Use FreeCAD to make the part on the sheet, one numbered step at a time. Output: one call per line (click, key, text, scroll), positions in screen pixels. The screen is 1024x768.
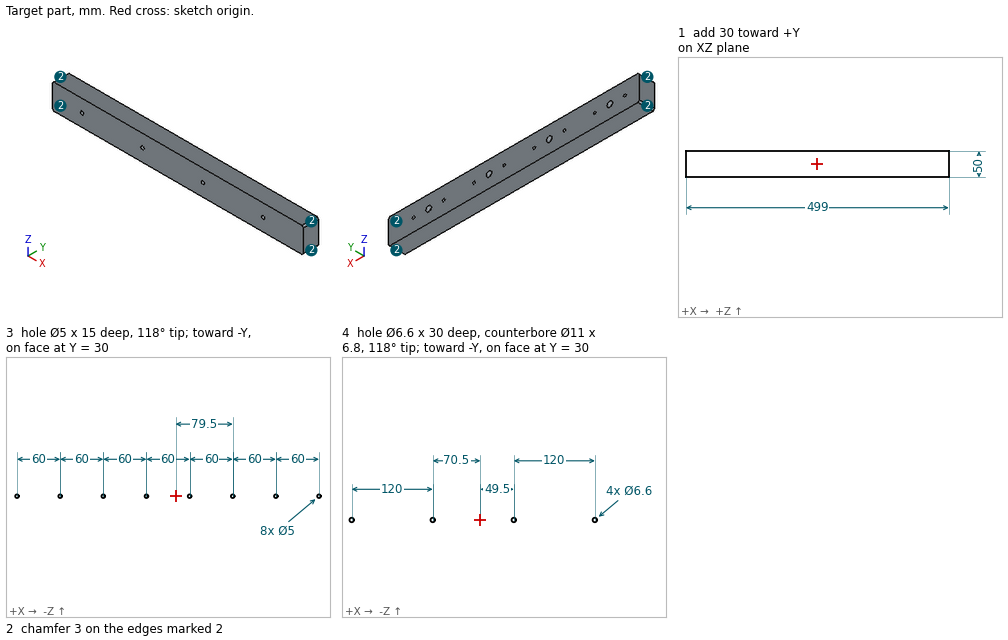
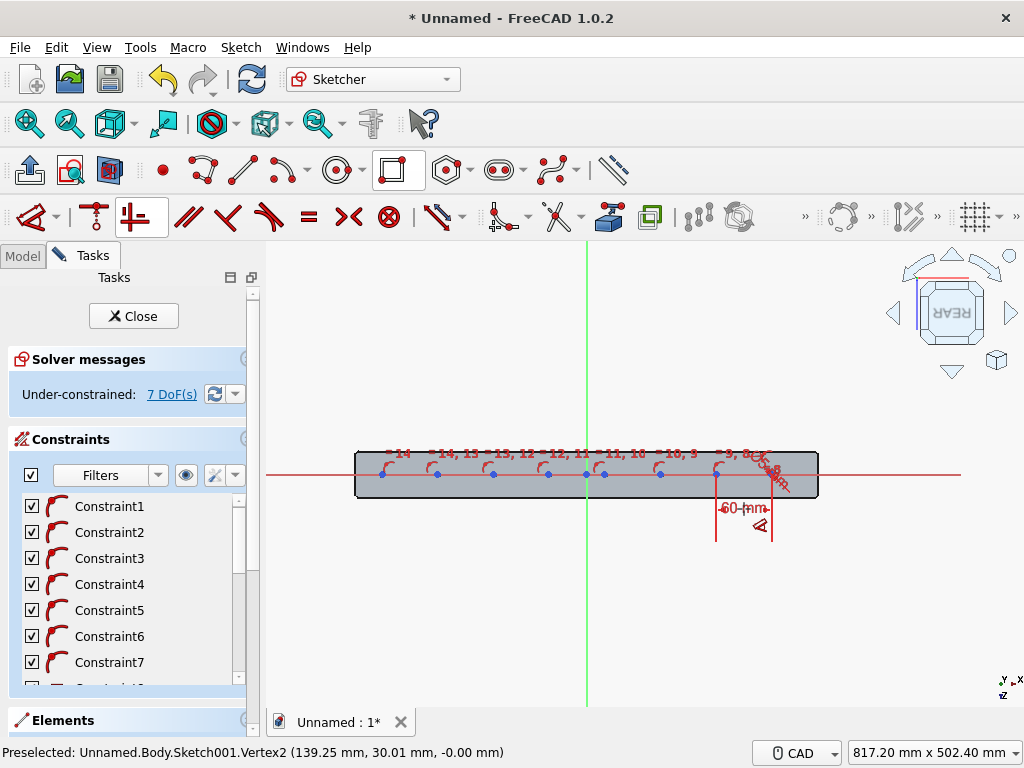
click(716, 475)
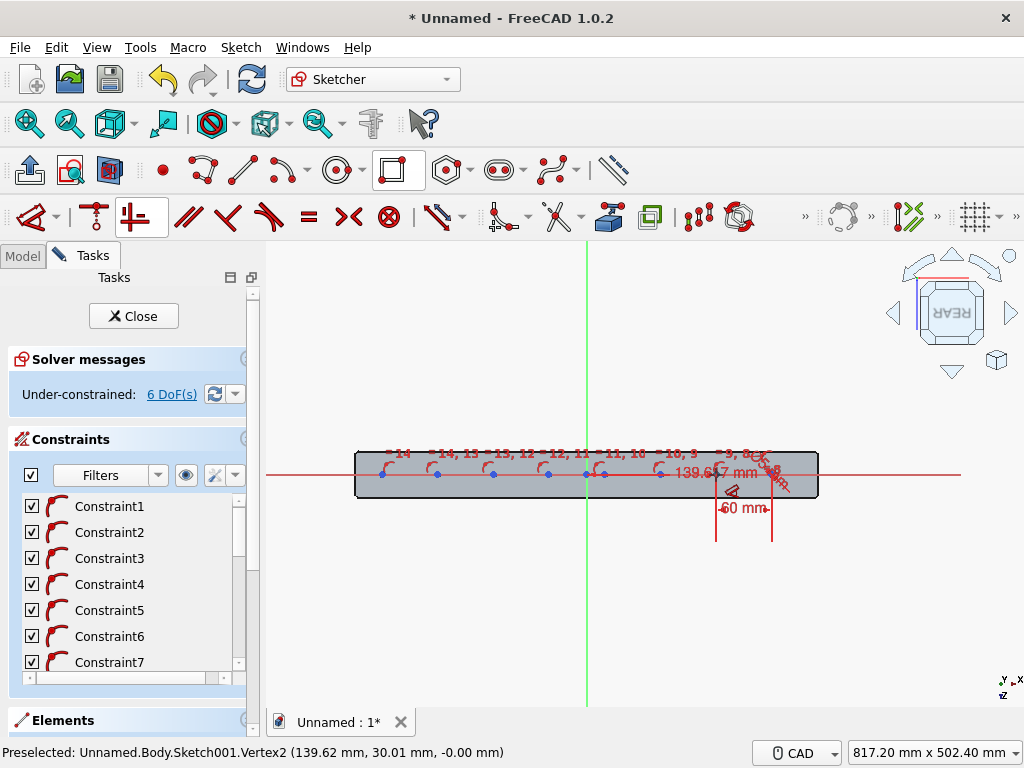
click(661, 475)
click(669, 509)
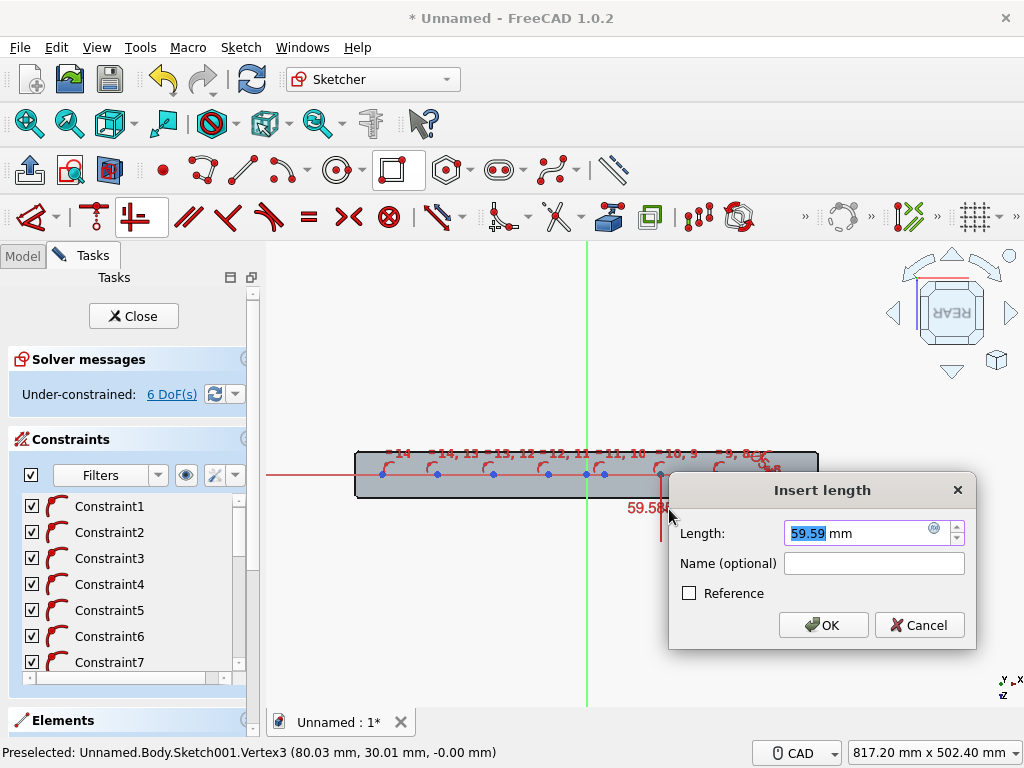
text(60)
key(Return)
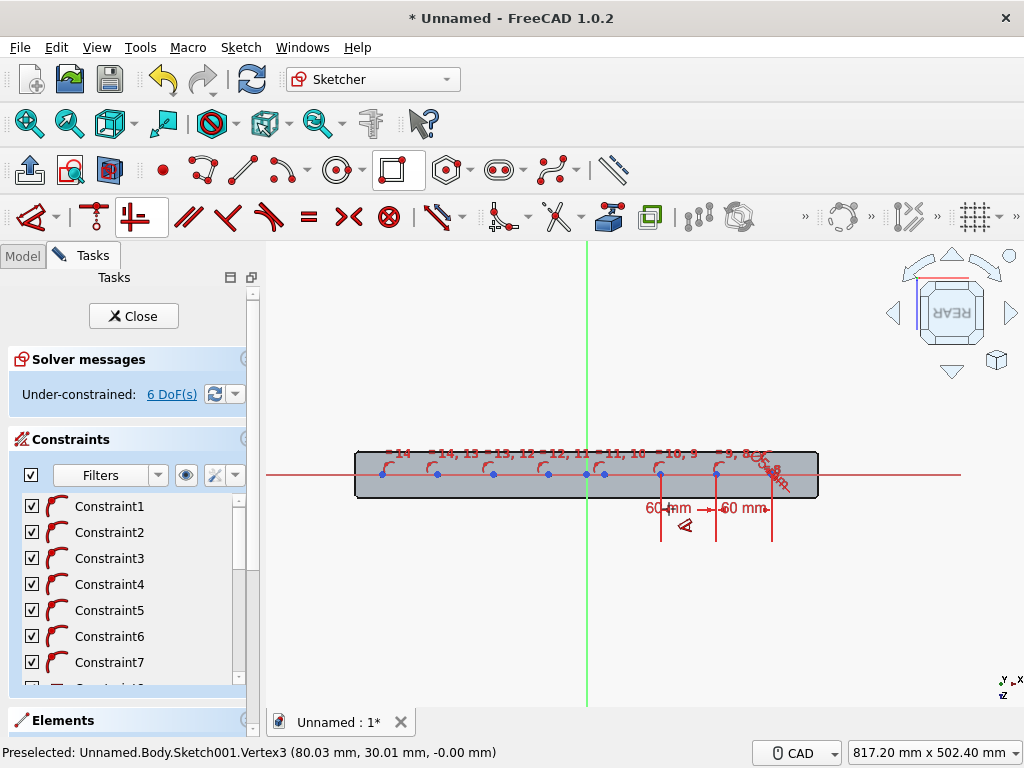
click(661, 475)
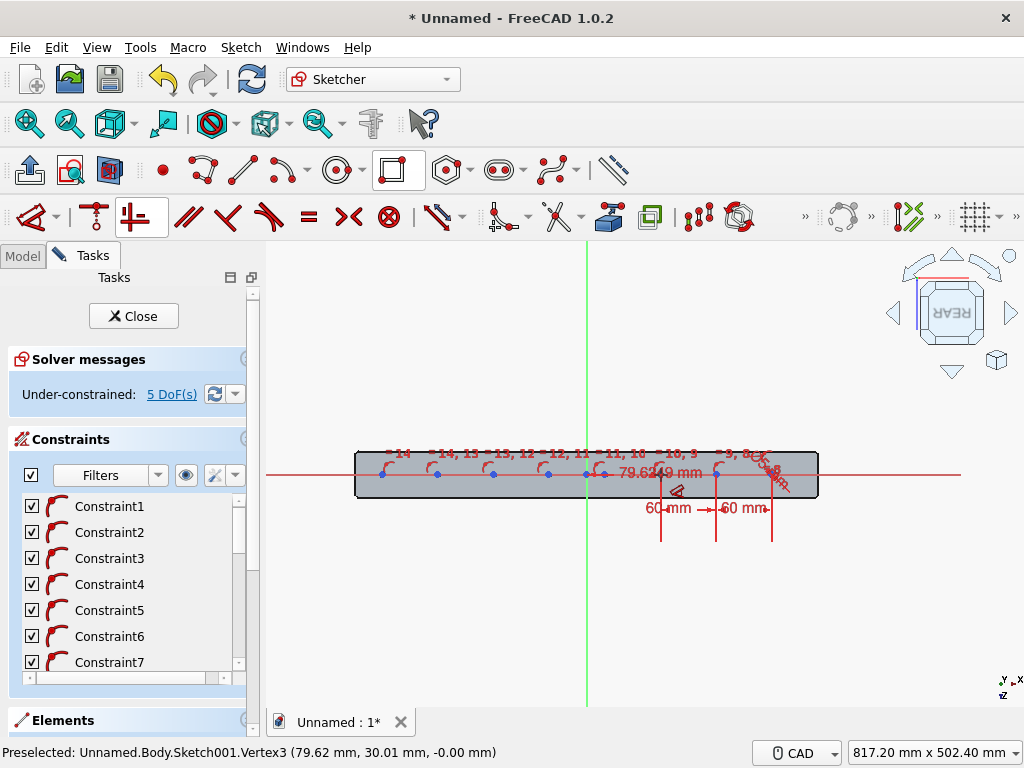
click(605, 475)
click(633, 441)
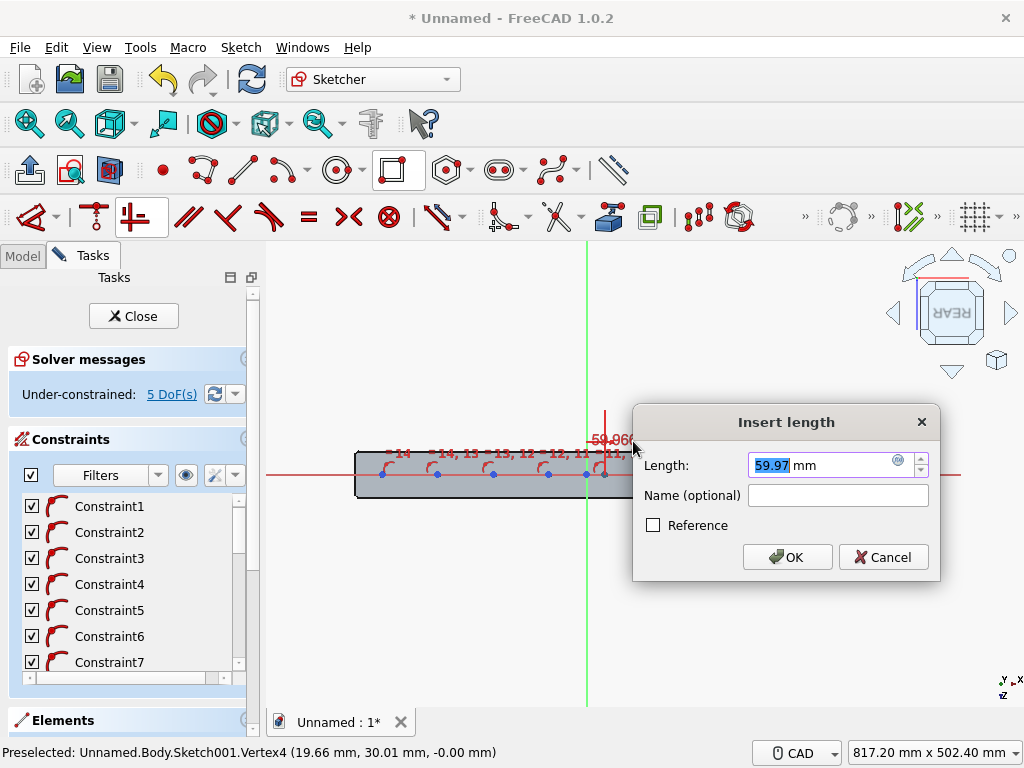
text(60)
key(Return)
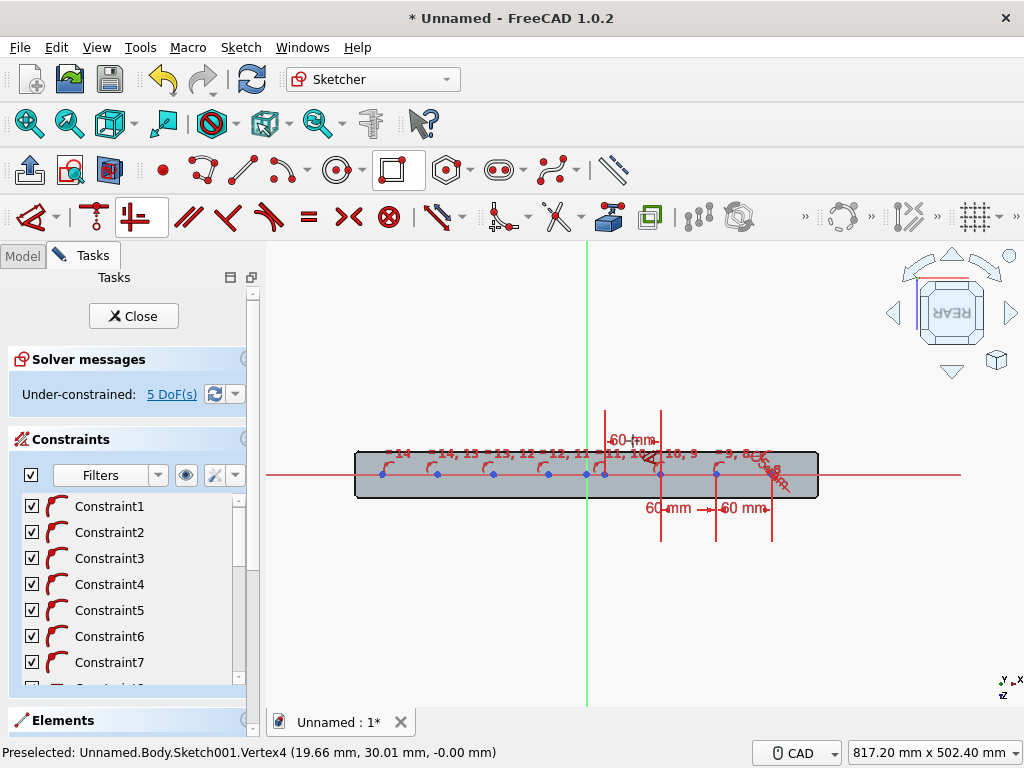
click(605, 475)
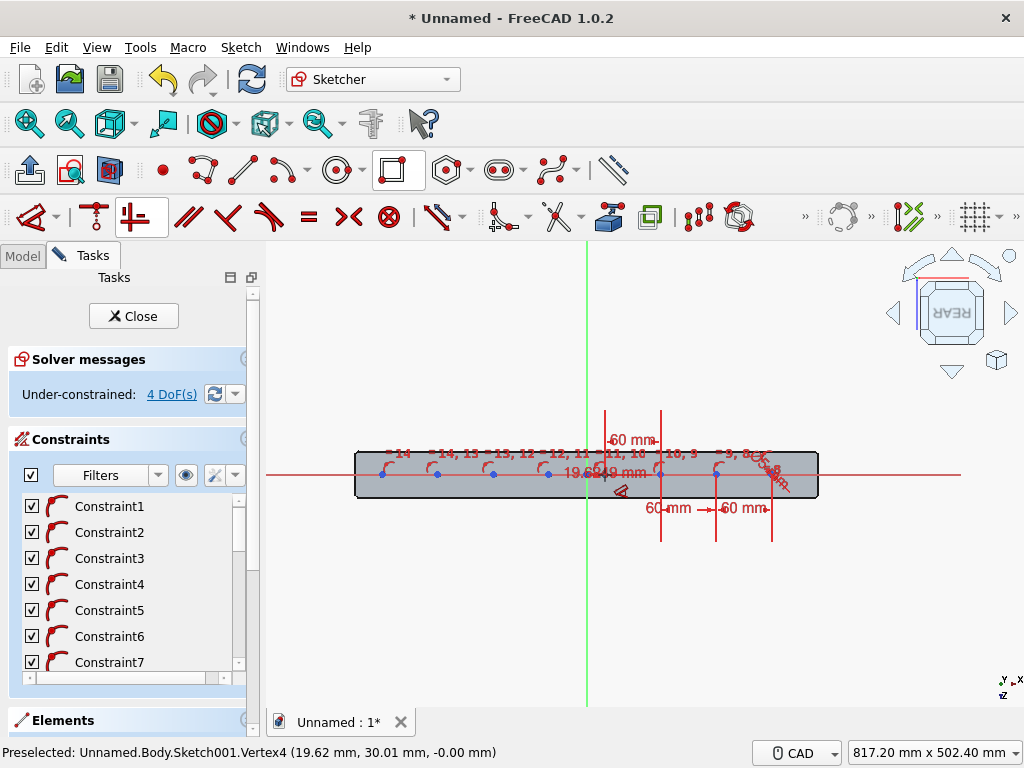
click(549, 475)
click(564, 509)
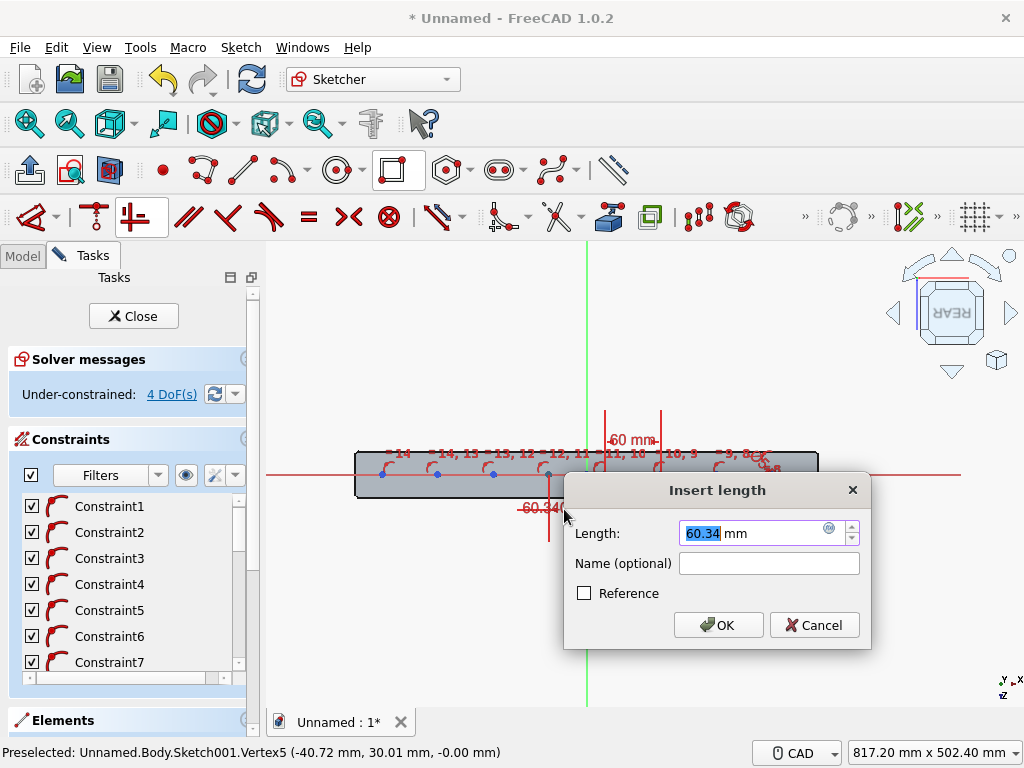
text(60)
key(Return)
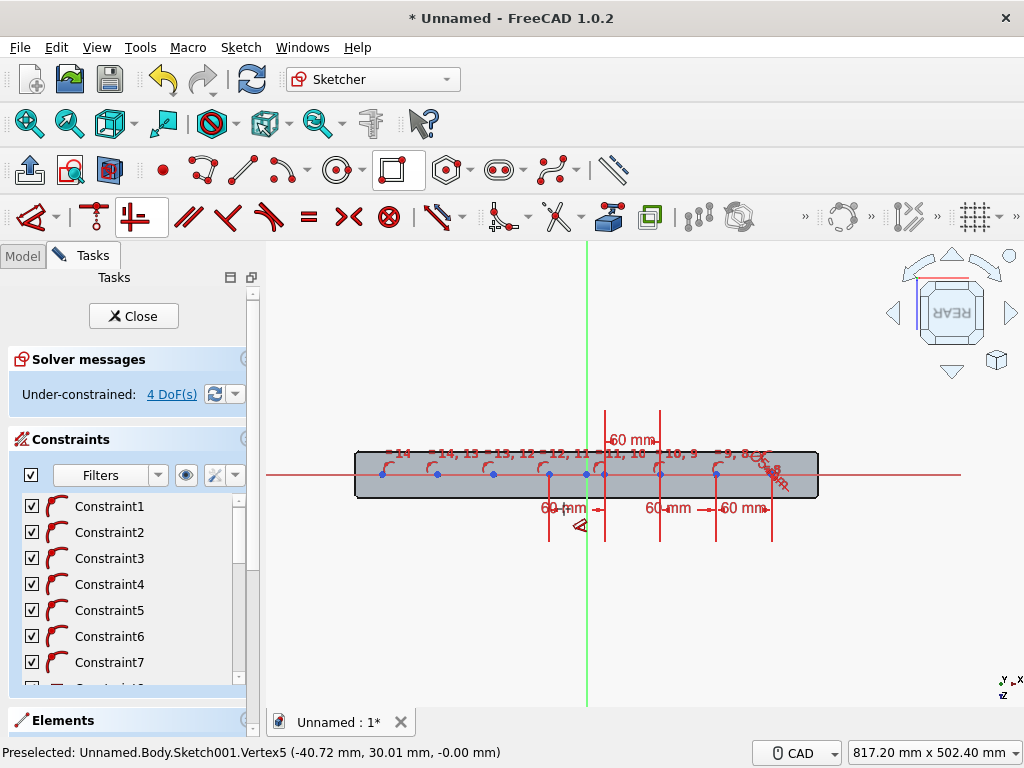
click(549, 475)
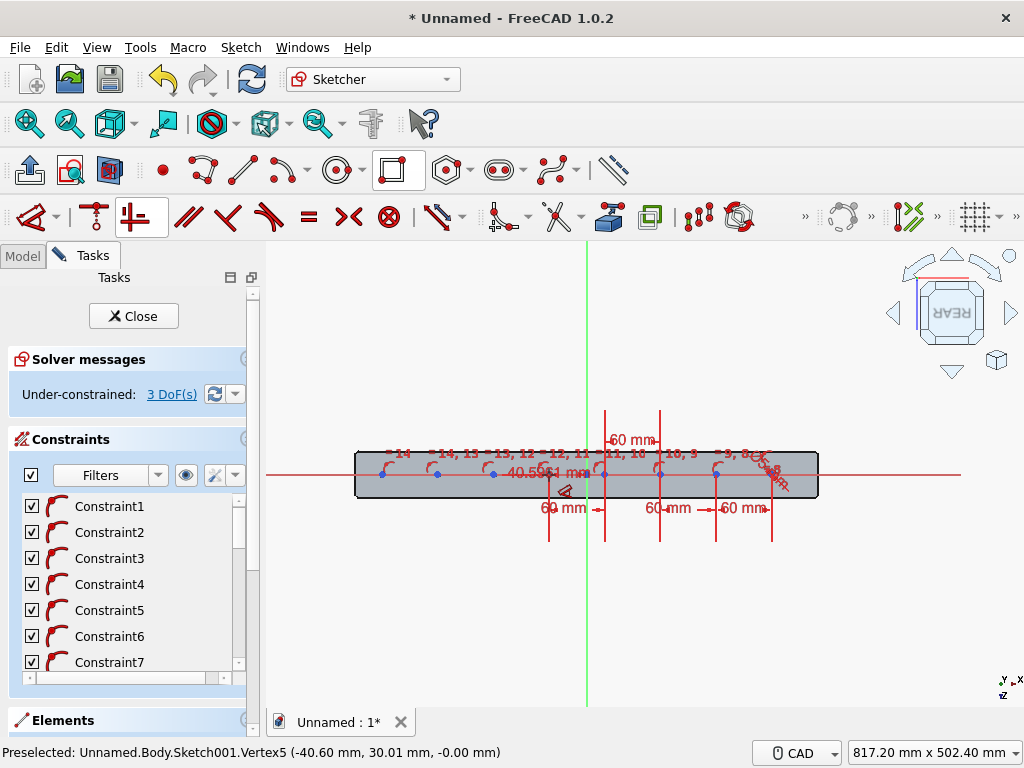
click(494, 475)
click(522, 441)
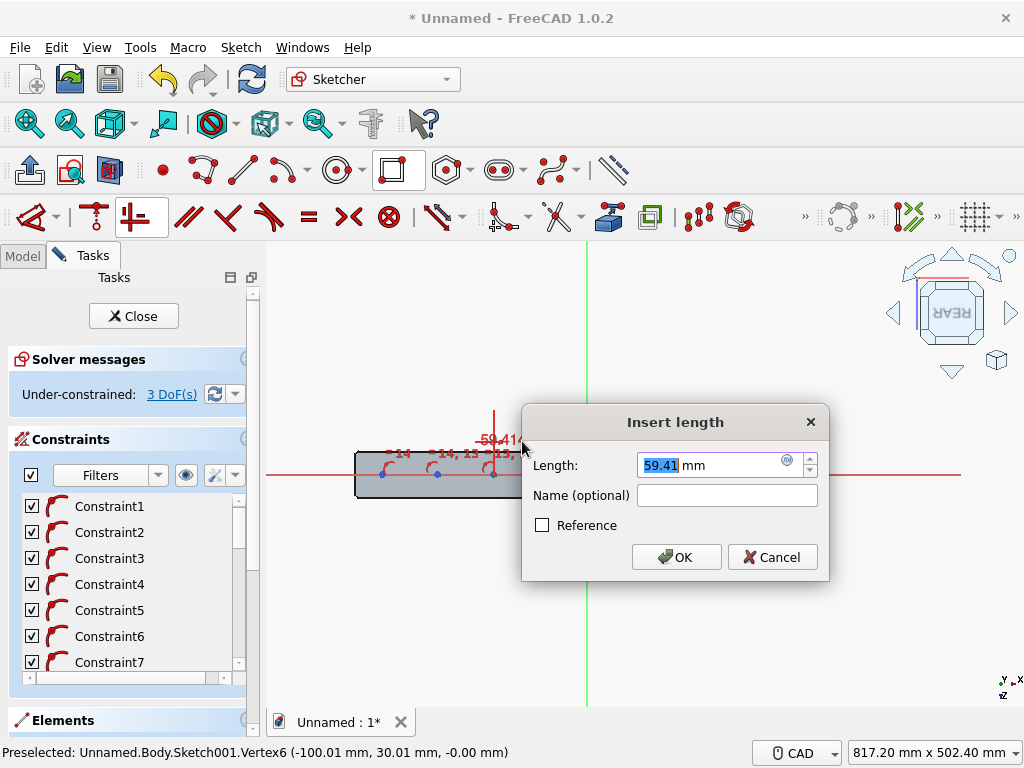
text(60)
key(Return)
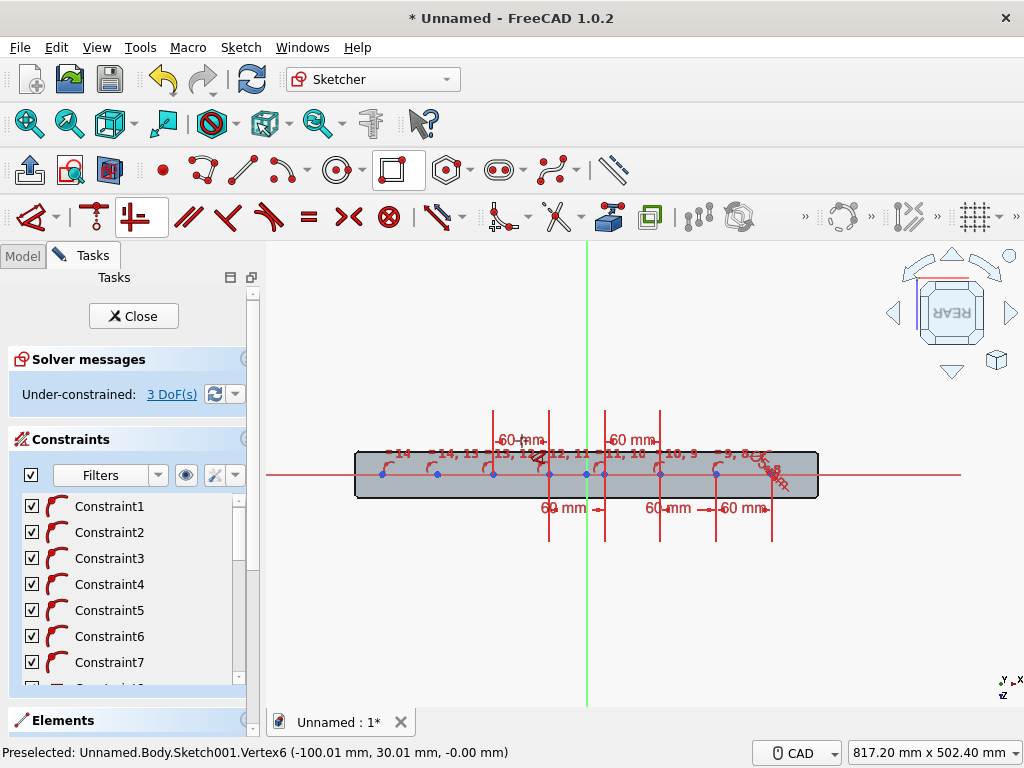
click(493, 475)